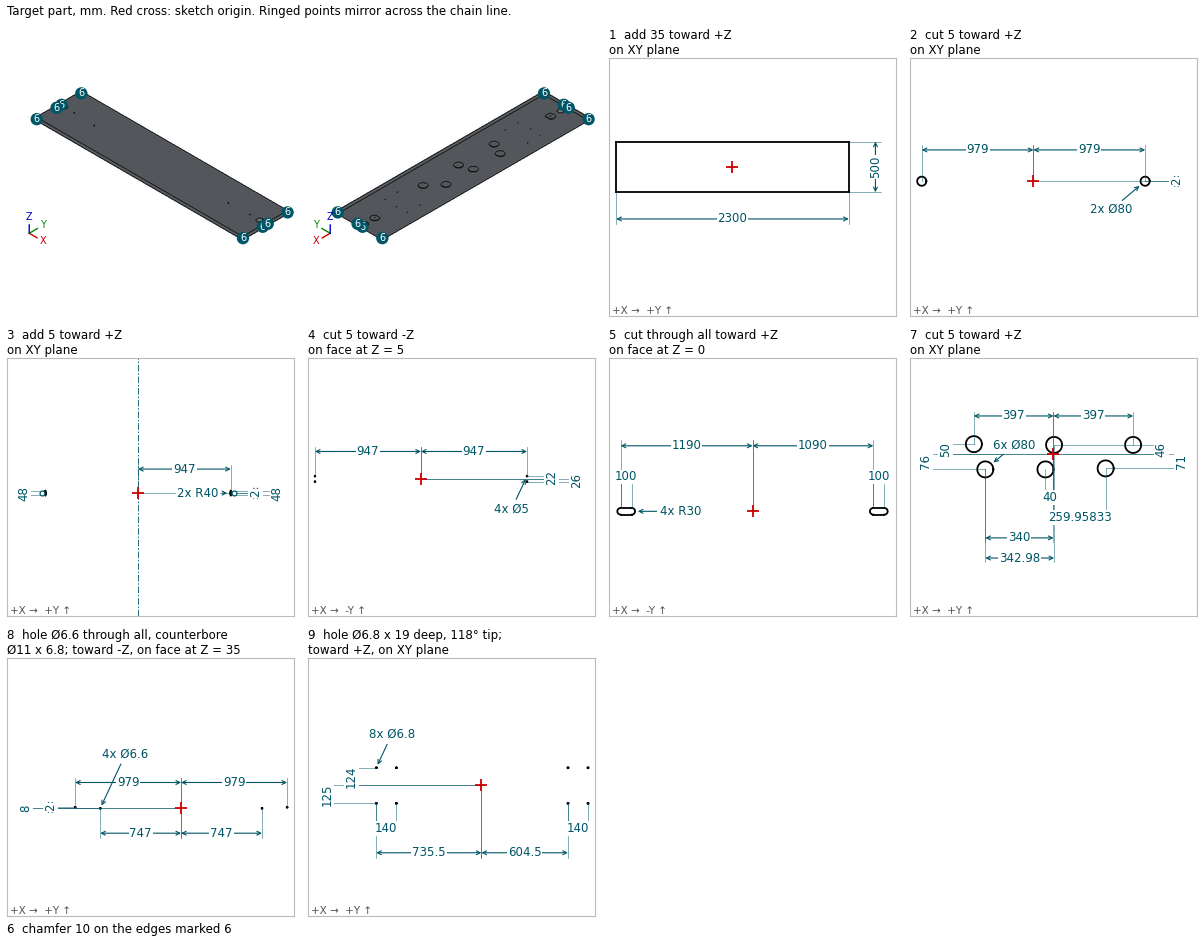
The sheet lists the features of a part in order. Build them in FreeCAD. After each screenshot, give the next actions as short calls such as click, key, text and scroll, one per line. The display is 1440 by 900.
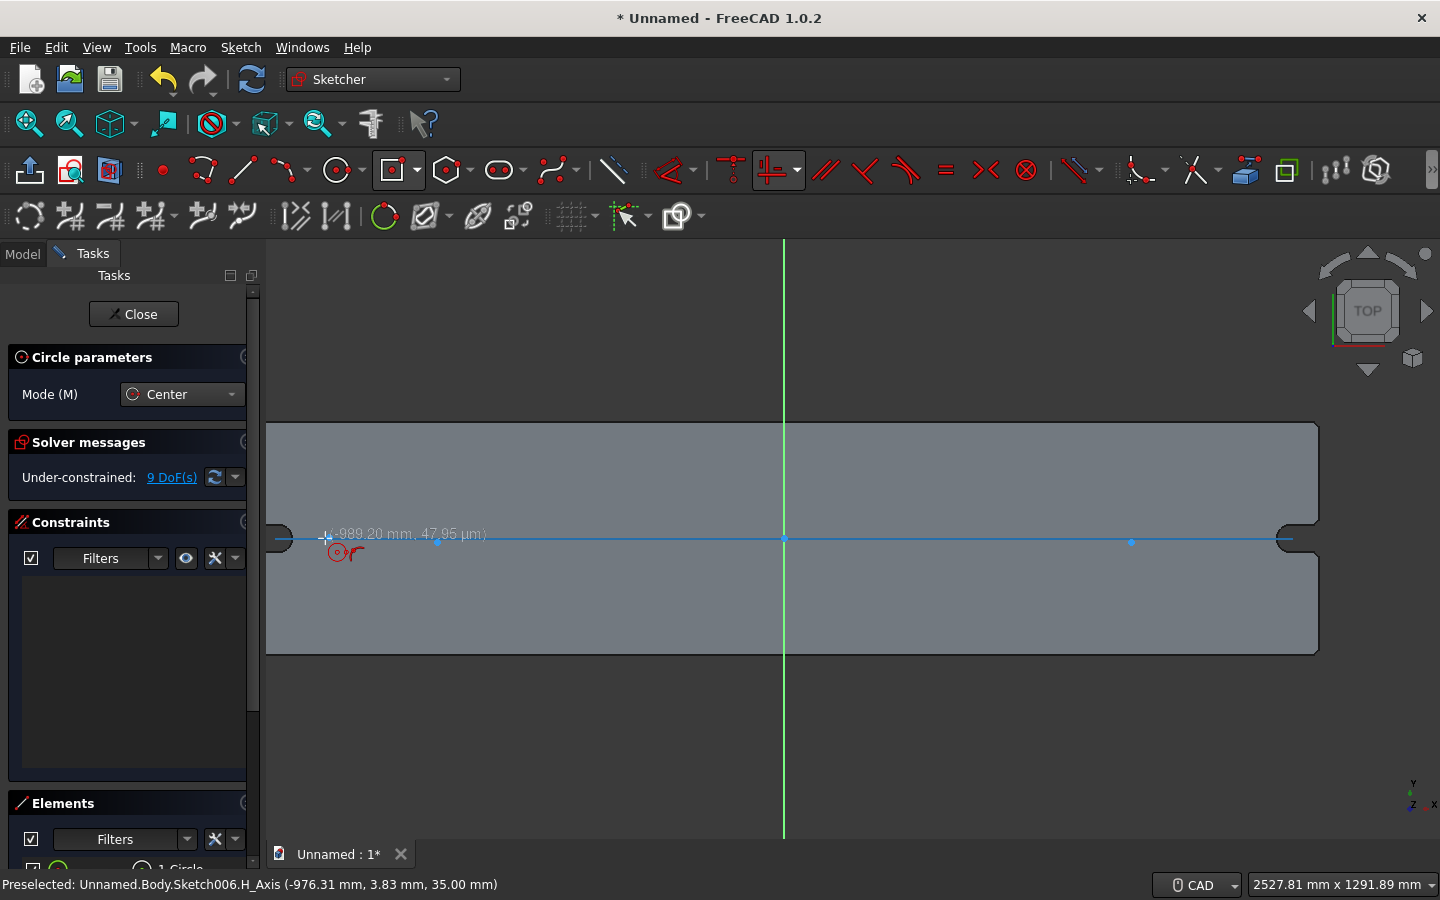
scroll(1239, 538, up, 15)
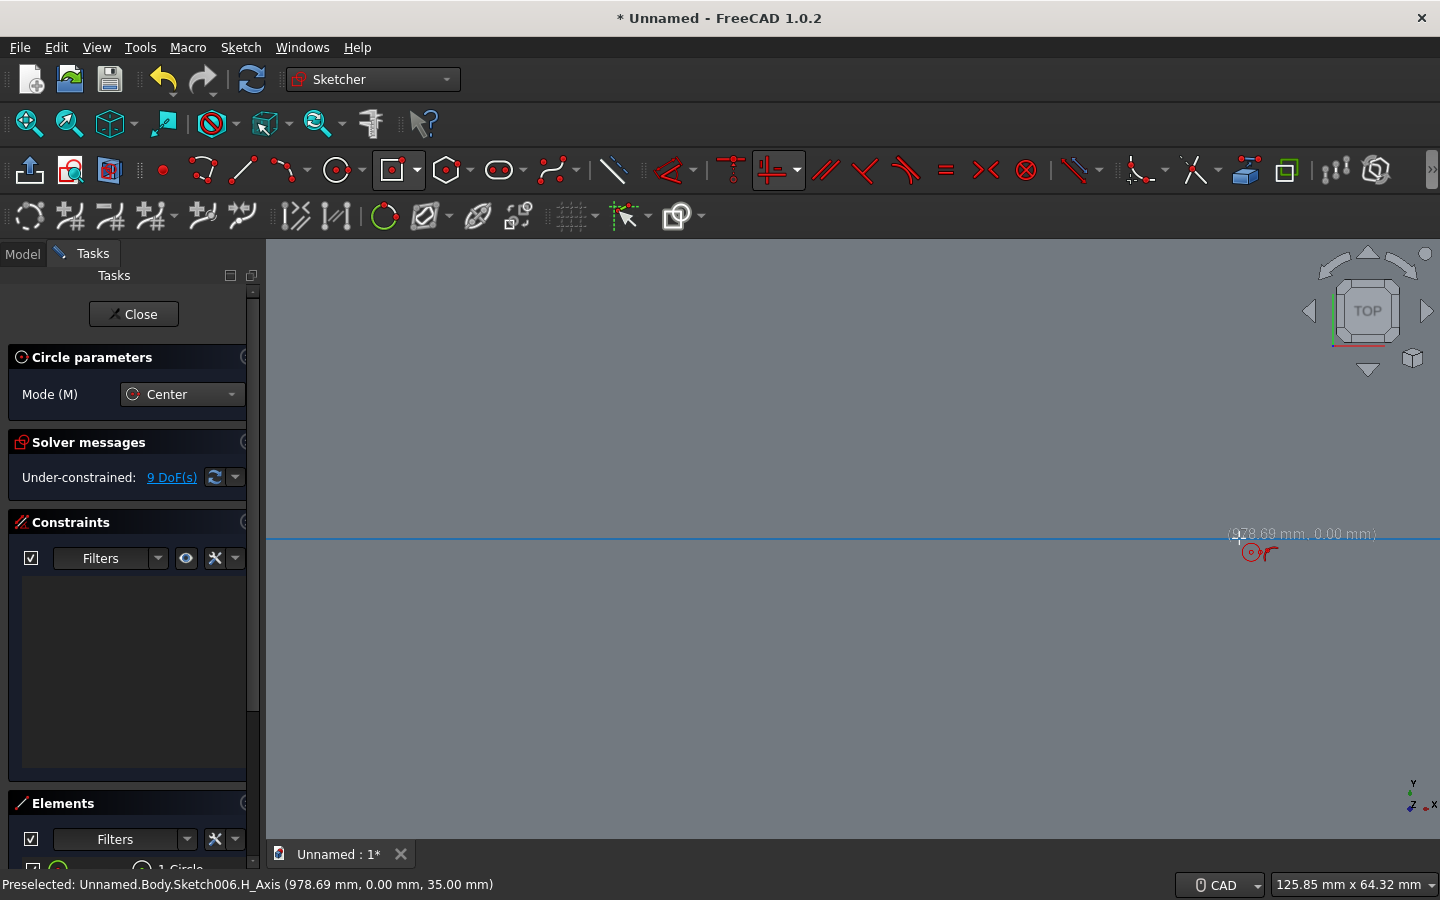
click(1226, 521)
click(1248, 499)
key(Escape)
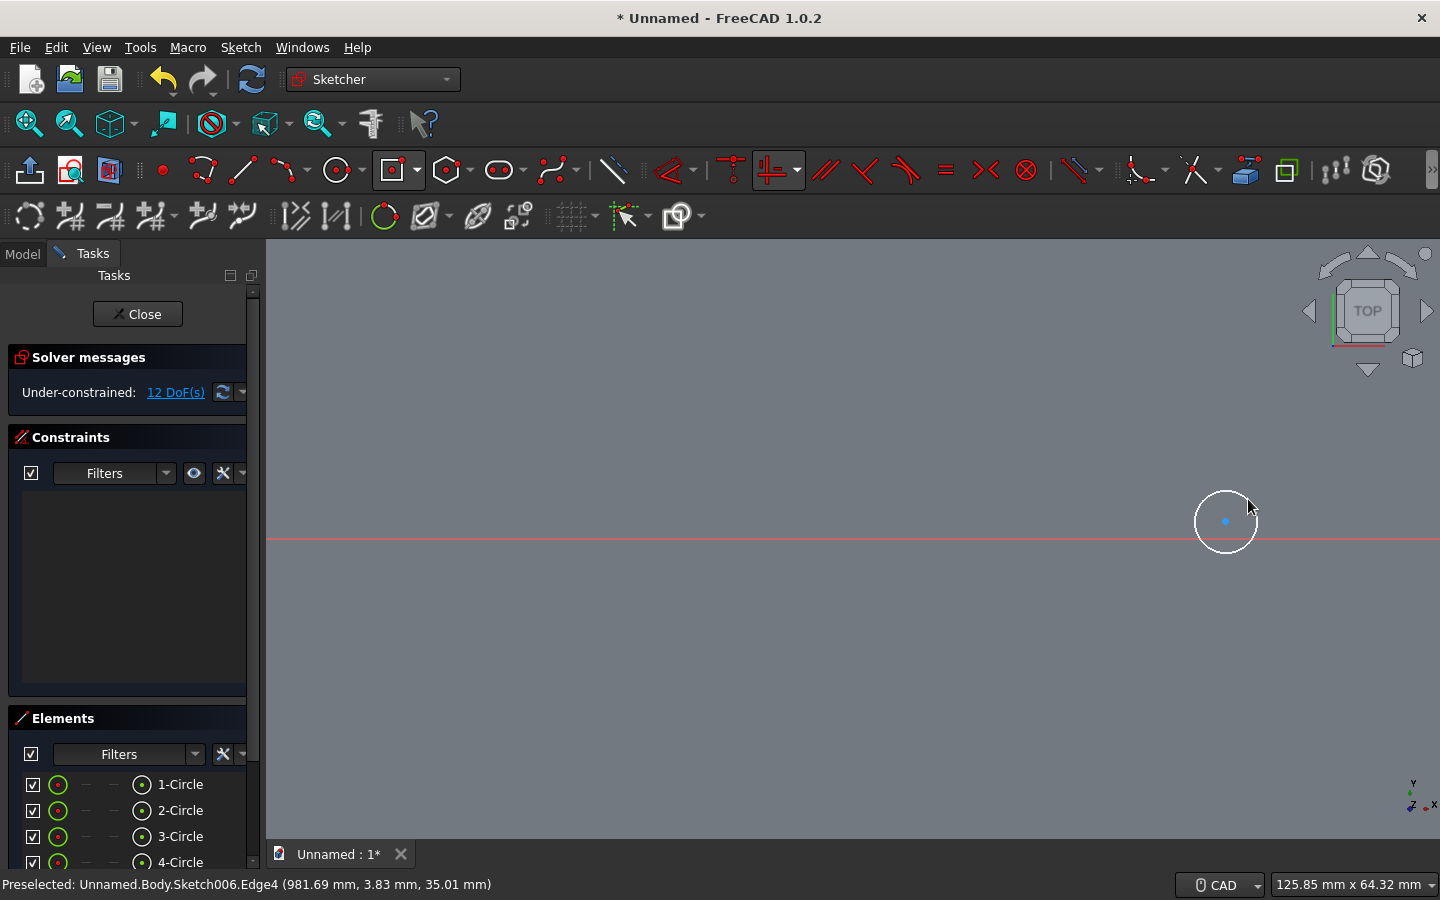
scroll(1240, 538, down, 15)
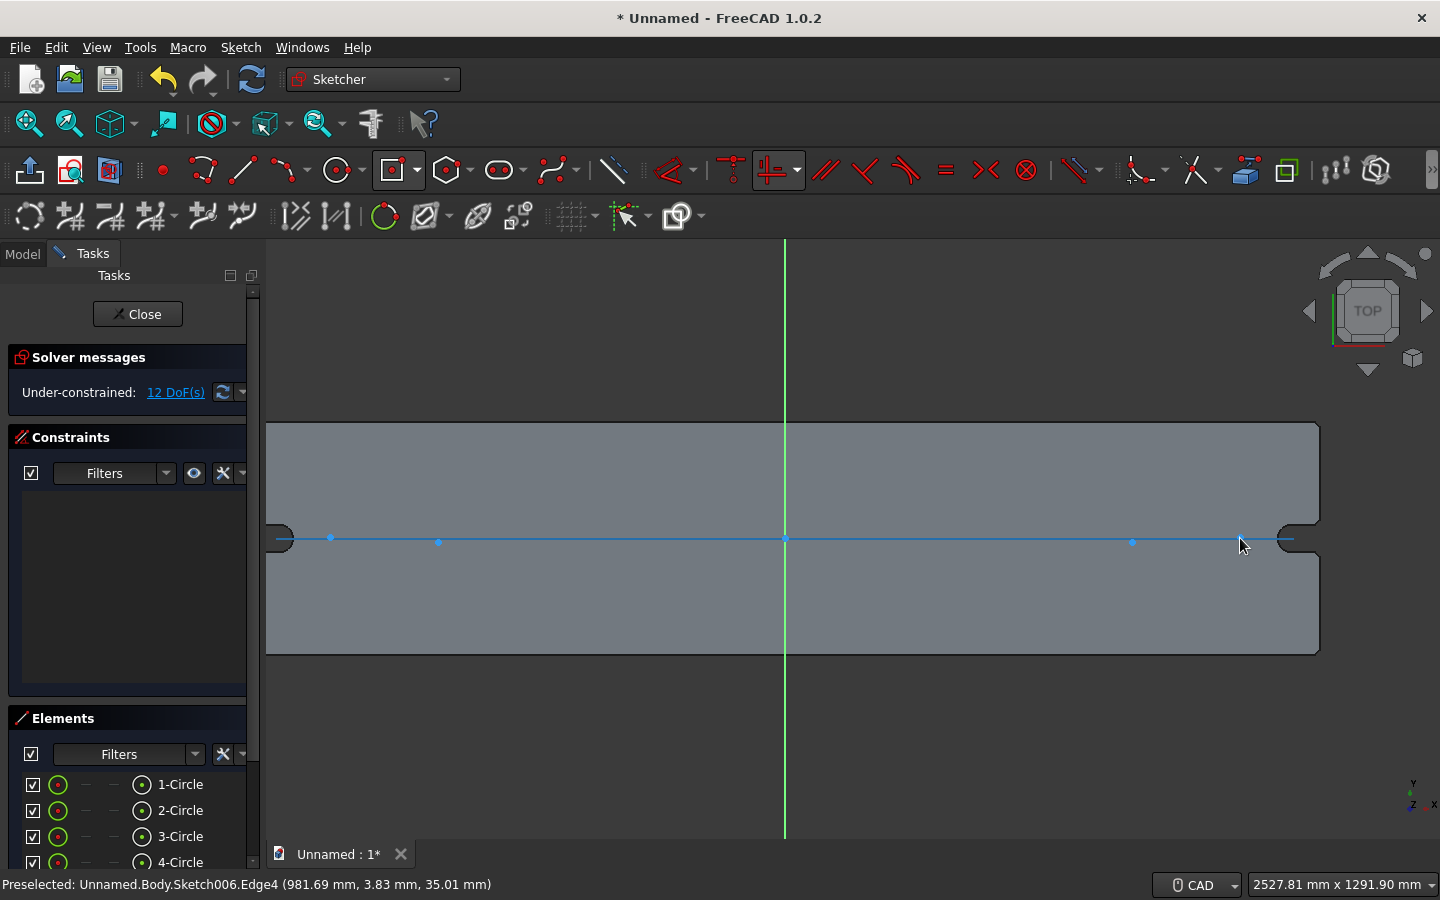
scroll(440, 541, up, 12)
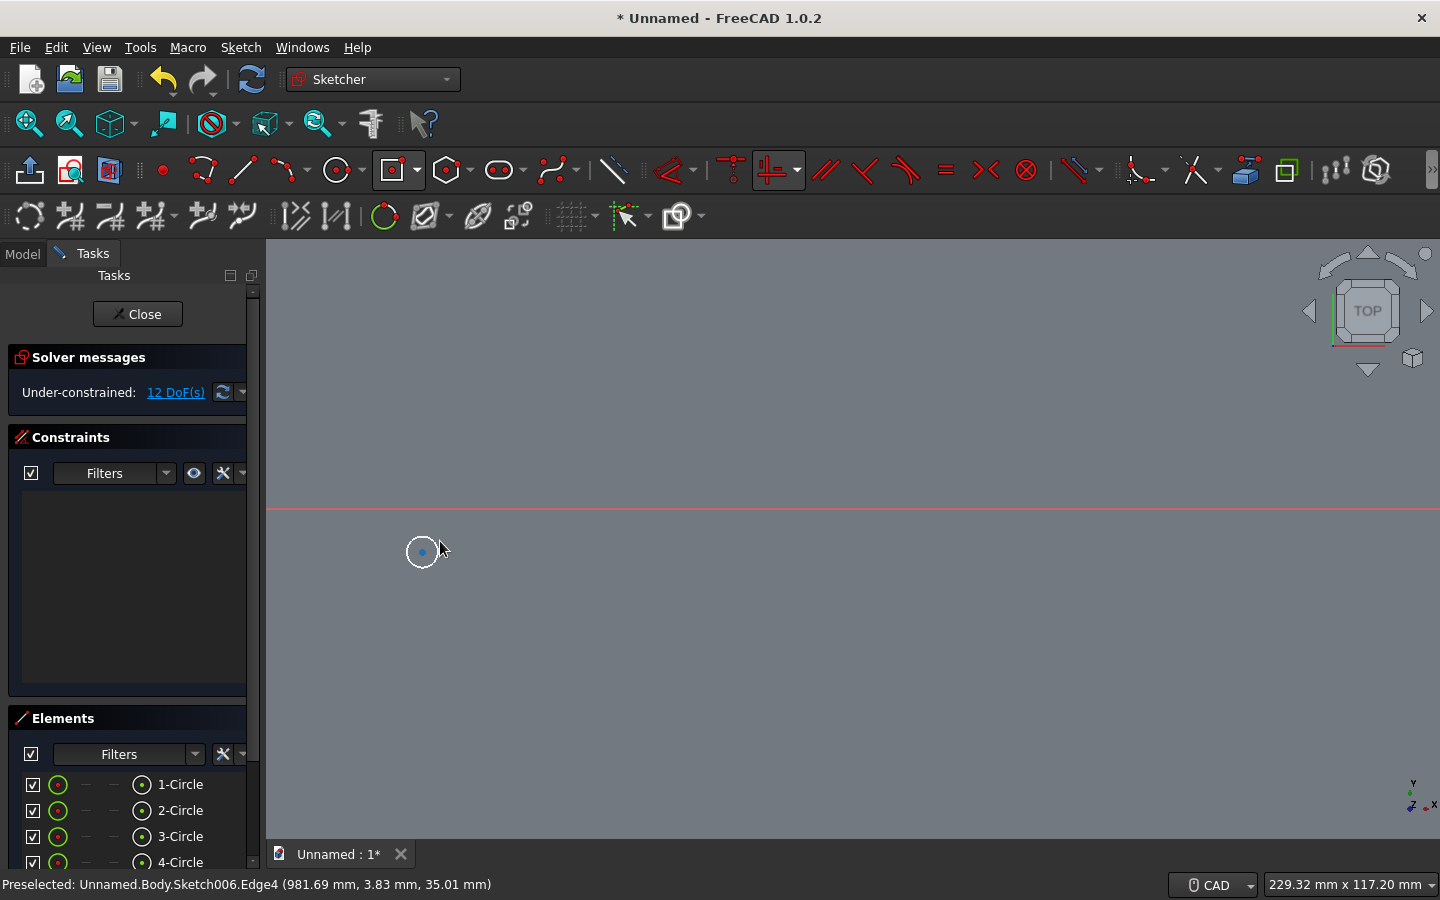
click(433, 541)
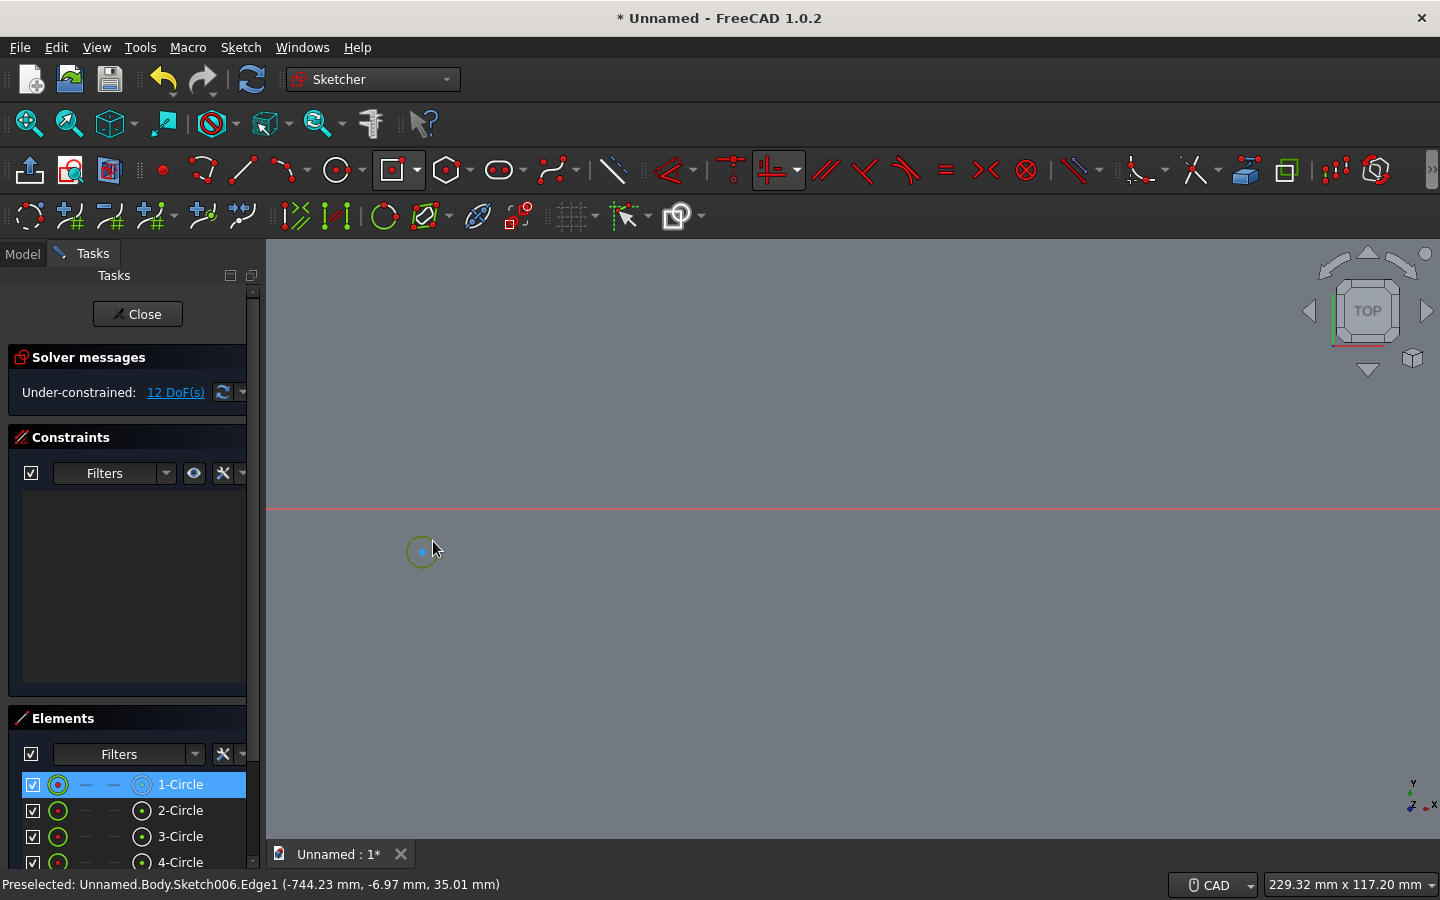
scroll(507, 540, down, 13)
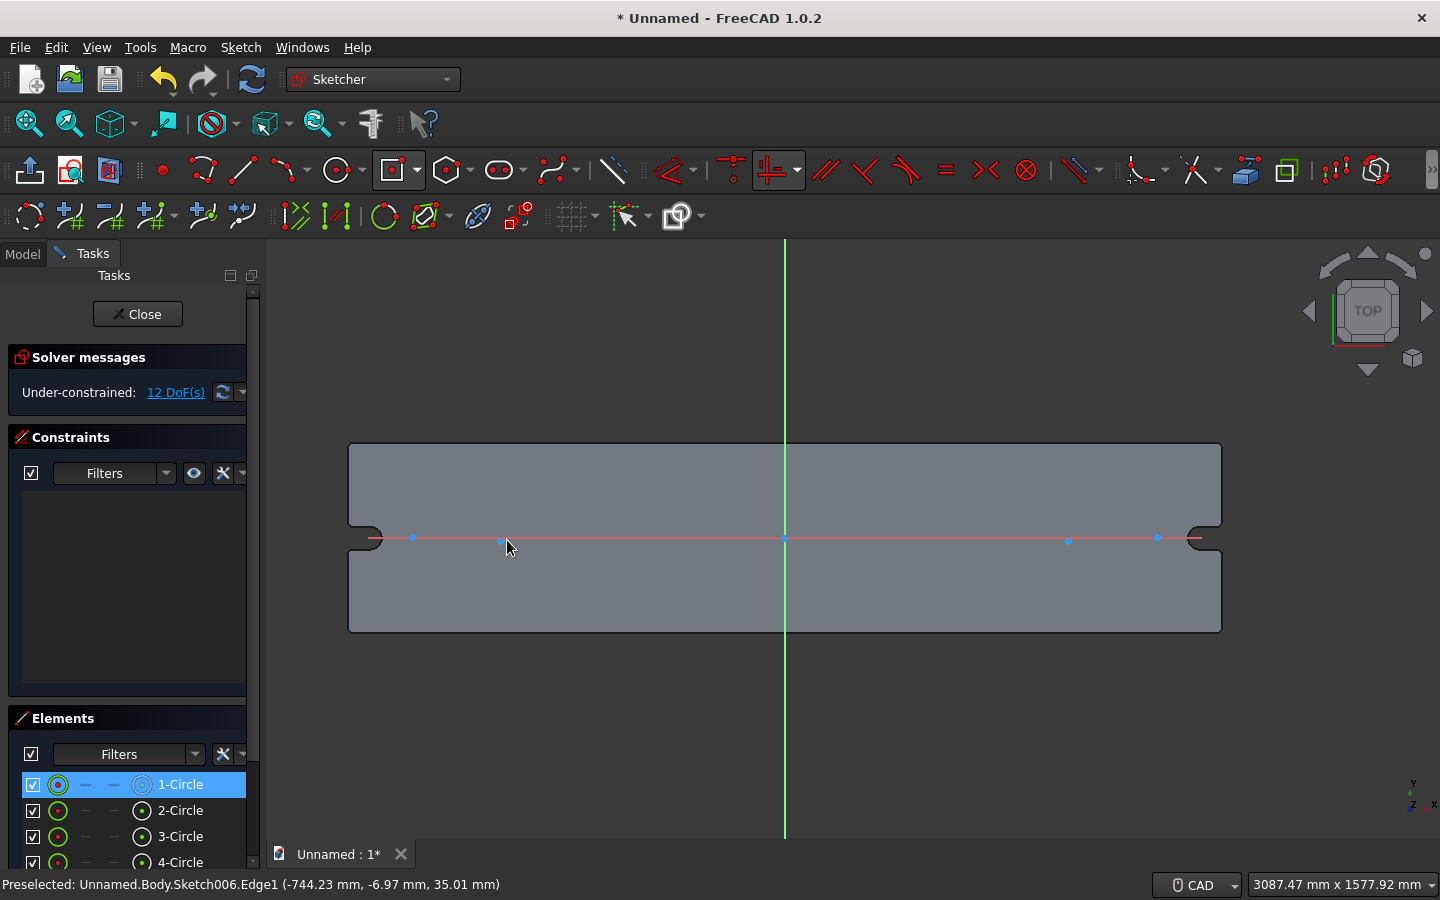
scroll(1070, 540, up, 13)